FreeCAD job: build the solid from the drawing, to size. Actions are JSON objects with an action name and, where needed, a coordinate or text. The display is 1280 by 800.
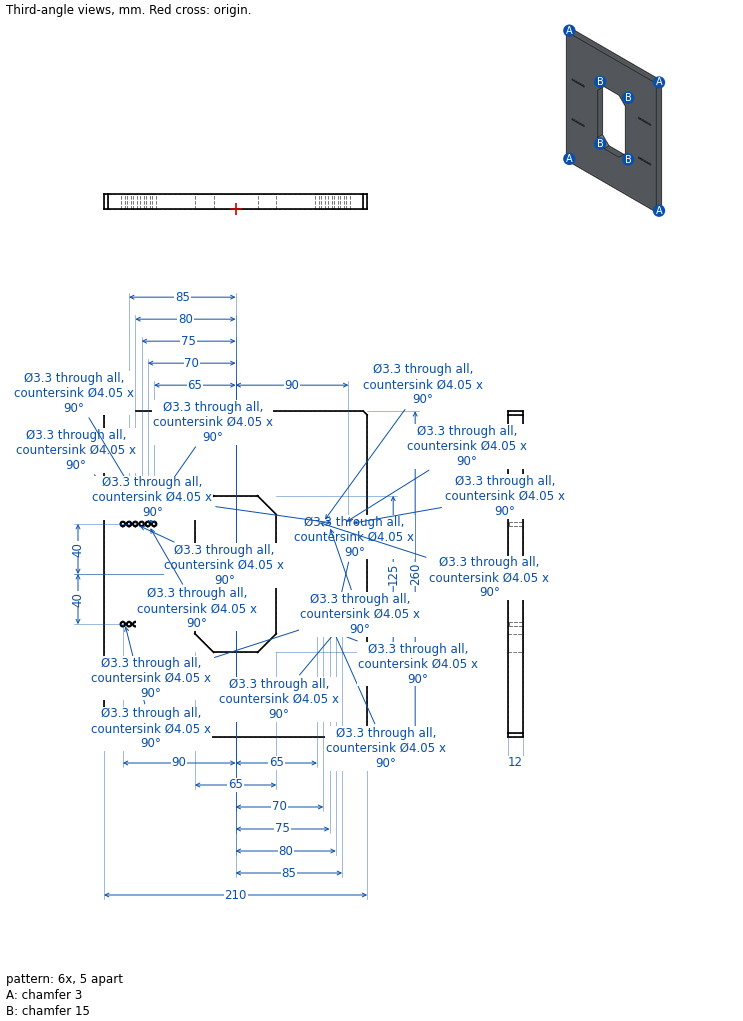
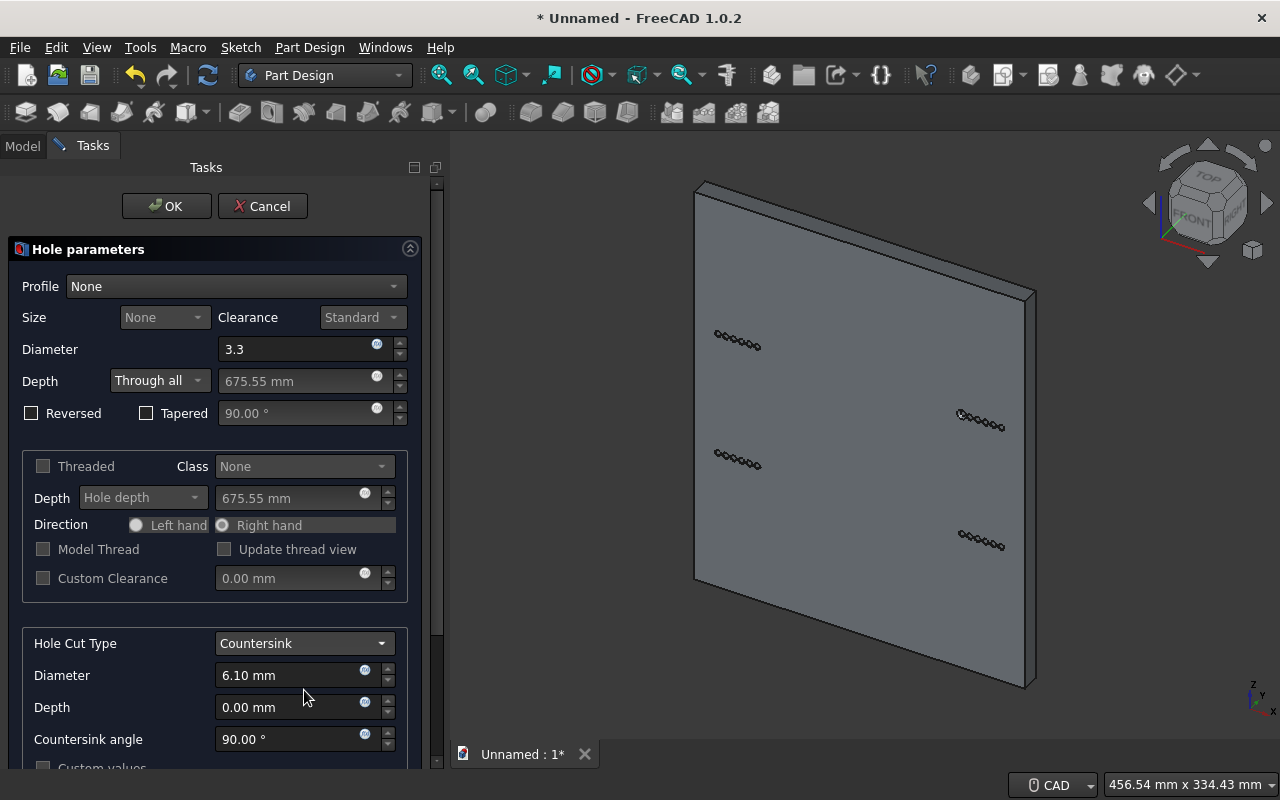
{"action": "triple_click", "coordinate": [298, 675]}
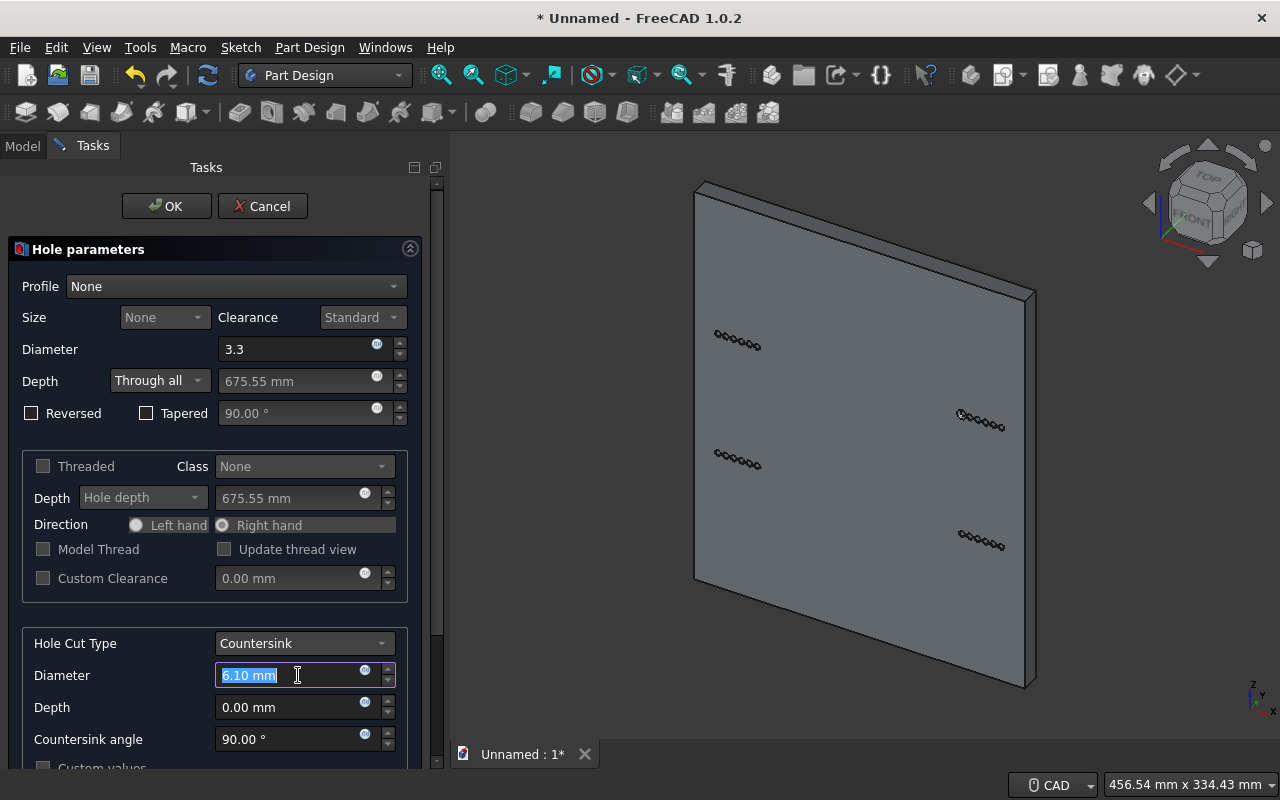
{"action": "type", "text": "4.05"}
{"action": "key", "text": "Tab"}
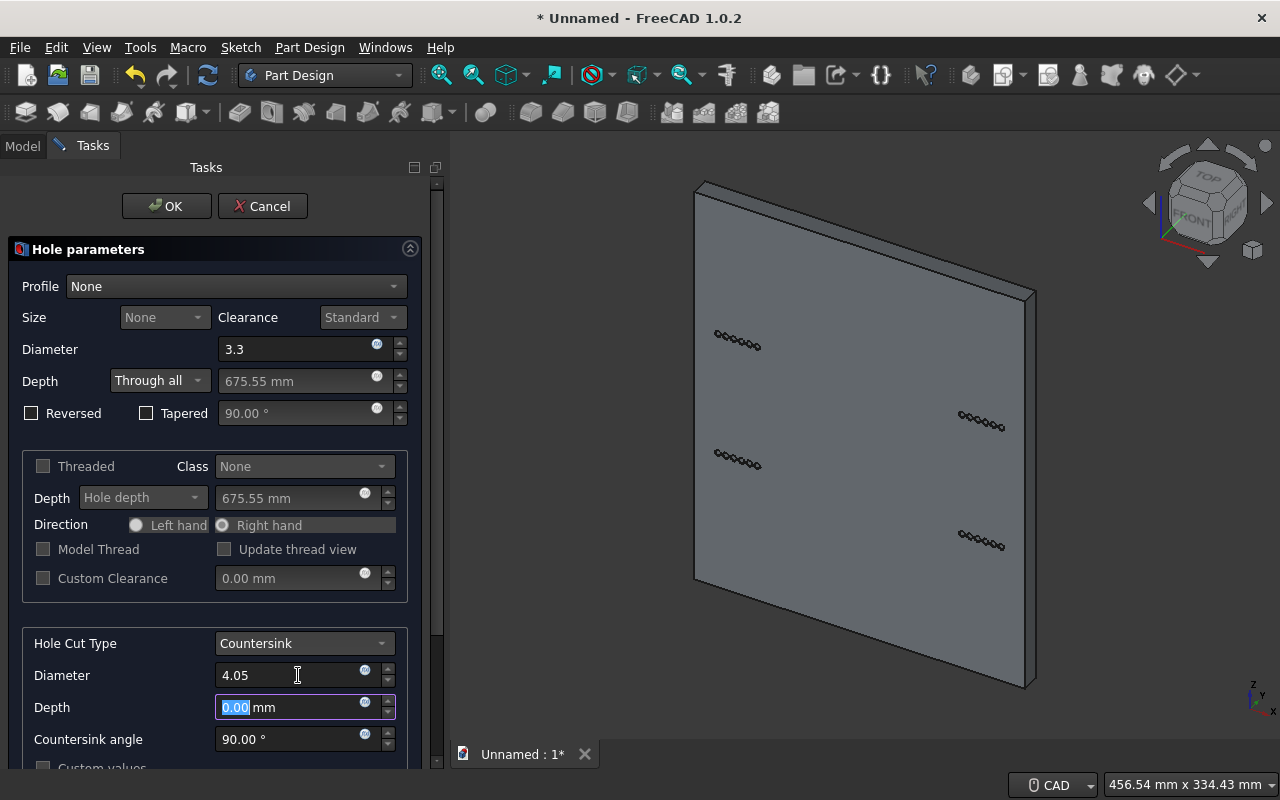
{"action": "left_click", "coordinate": [167, 206]}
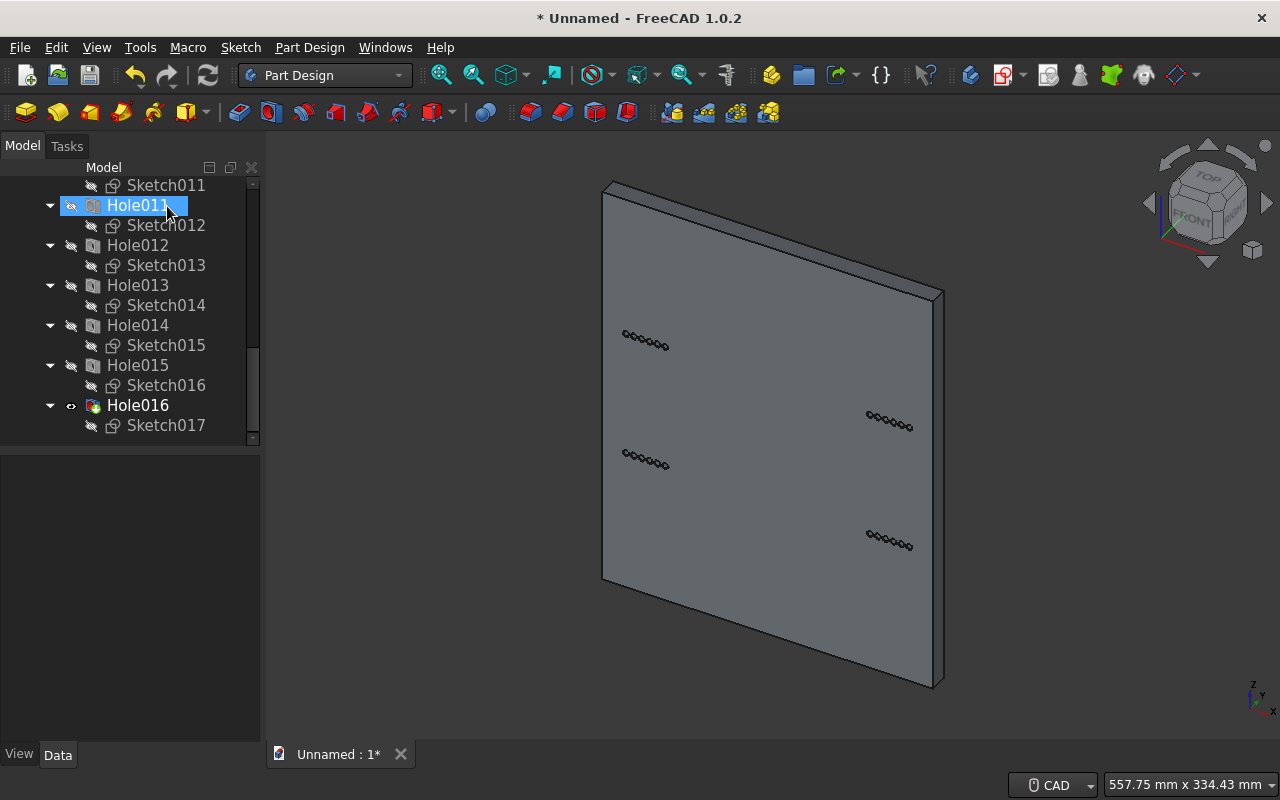
{"action": "left_click", "coordinate": [938, 295]}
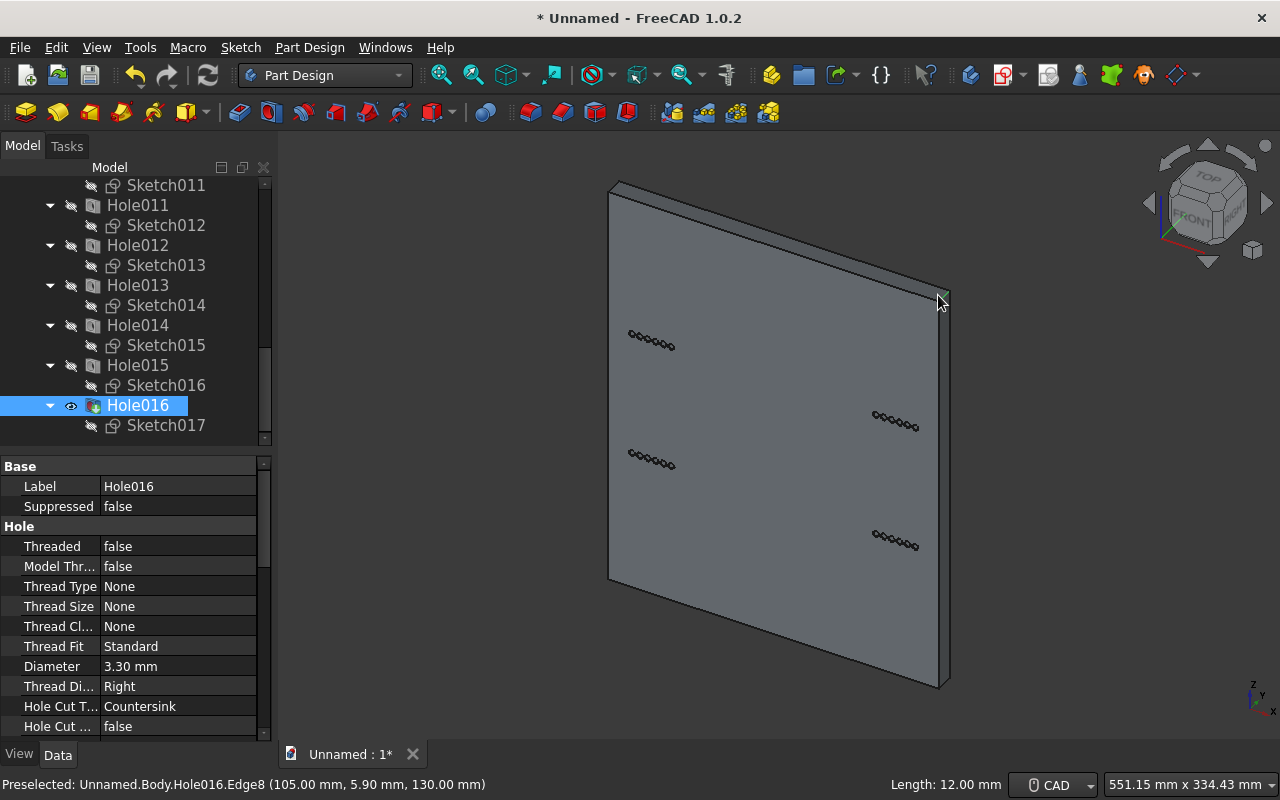
{"action": "scroll", "coordinate": [614, 186], "scroll_direction": "up", "scroll_amount": 4}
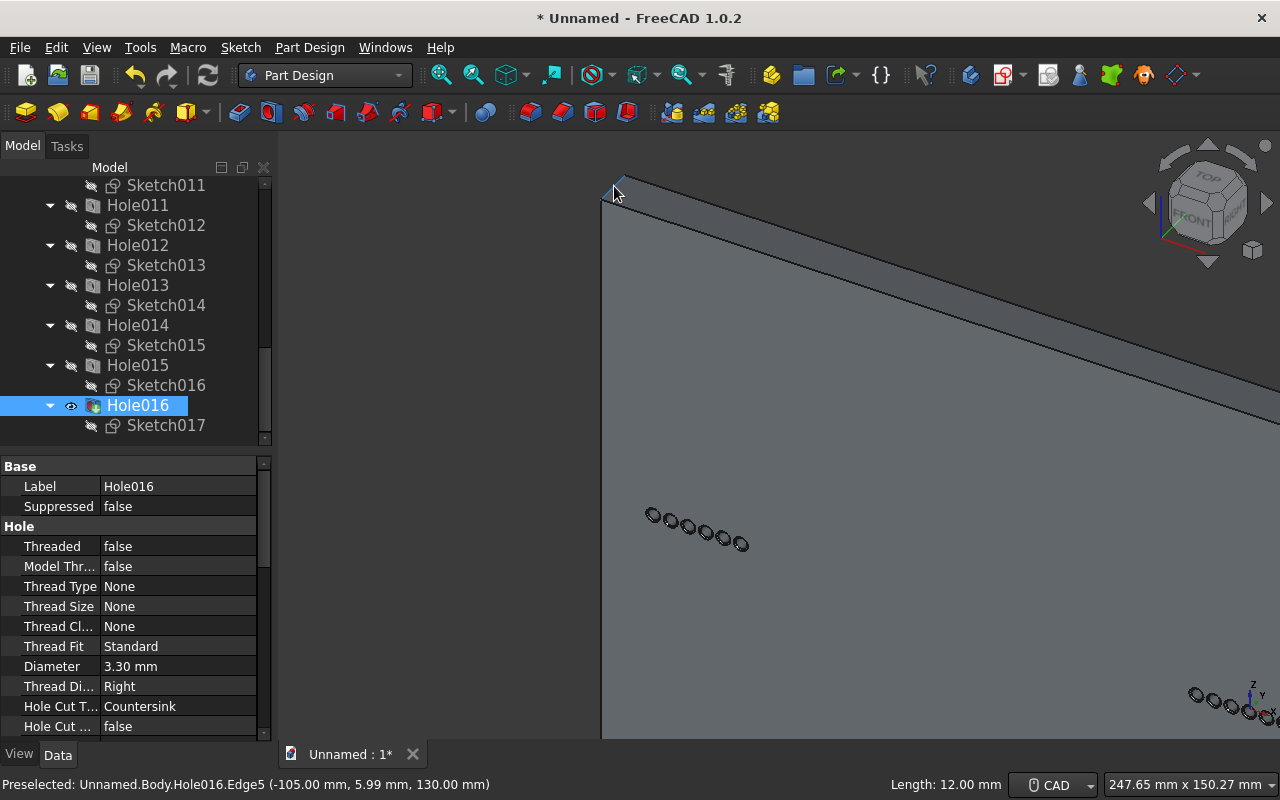
{"action": "left_click", "coordinate": [442, 76]}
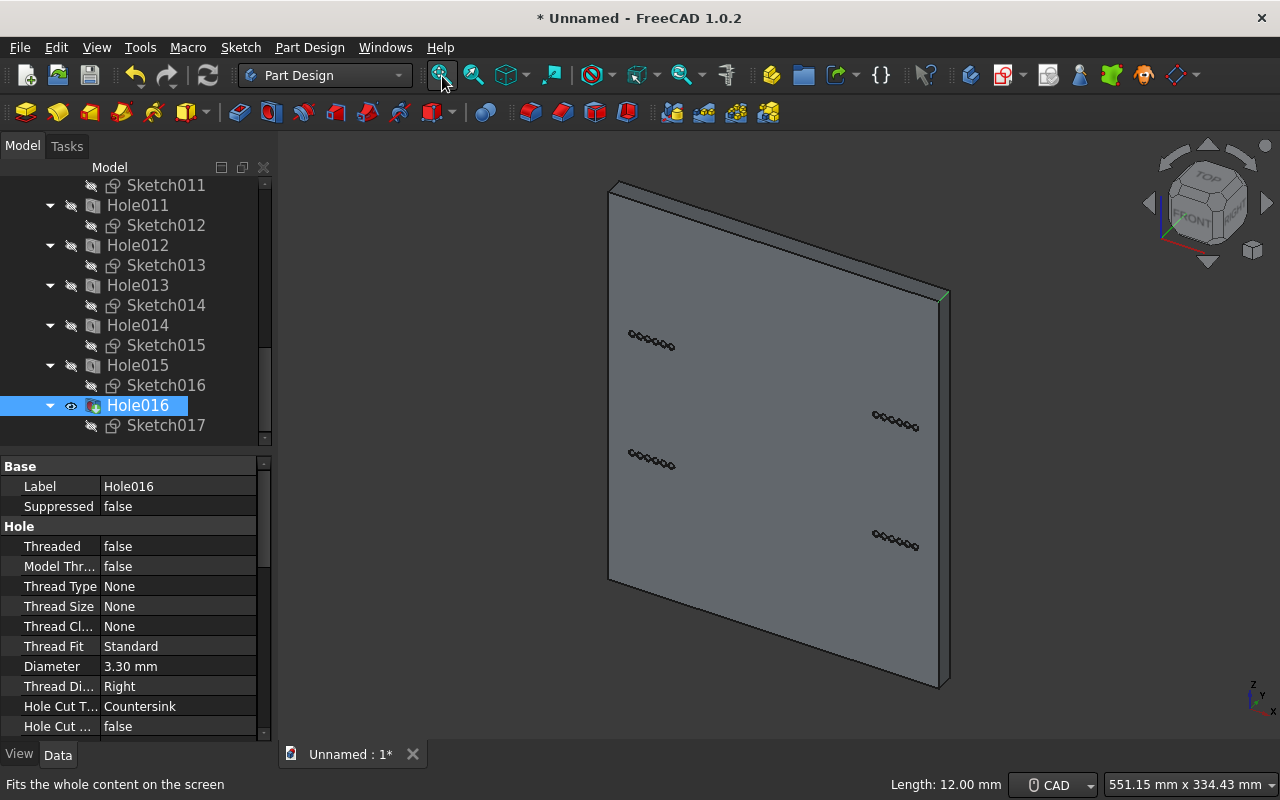
{"action": "key", "text": "0"}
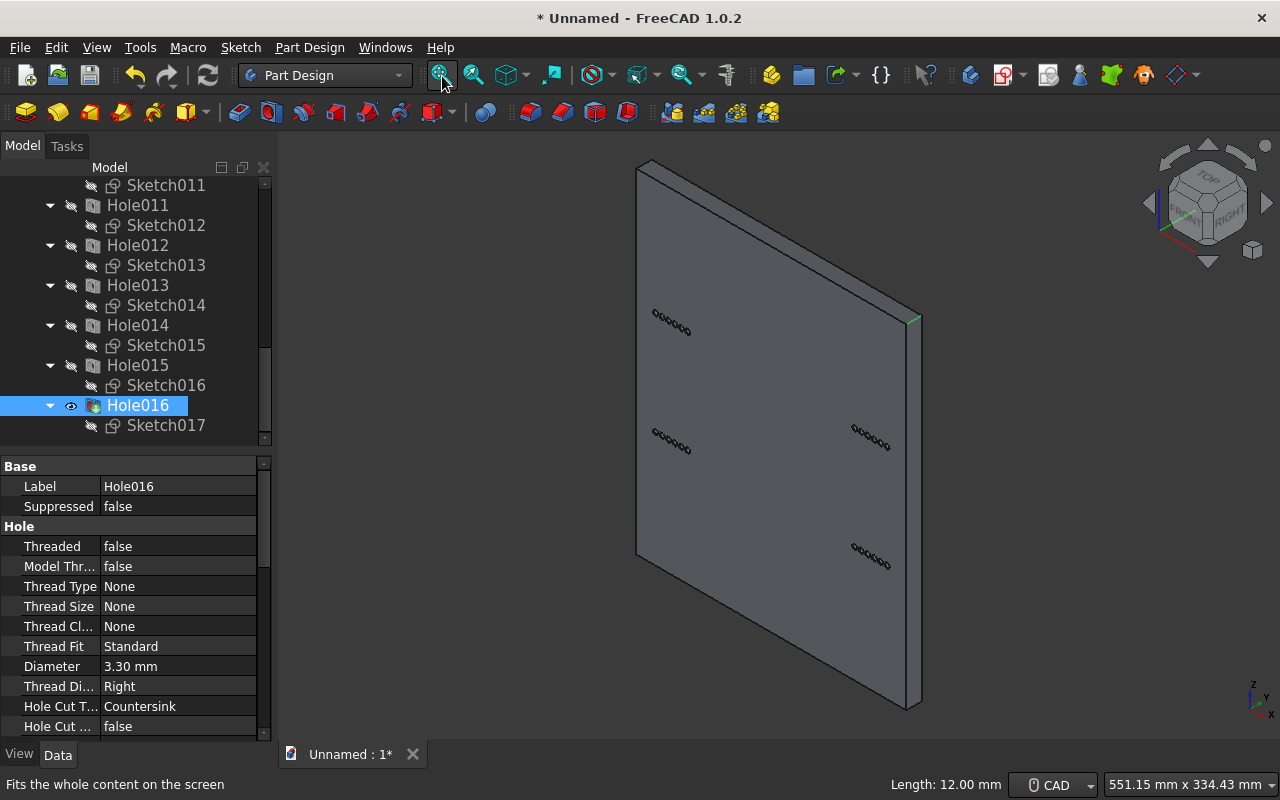
{"action": "scroll", "coordinate": [644, 163], "scroll_direction": "up", "scroll_amount": 4}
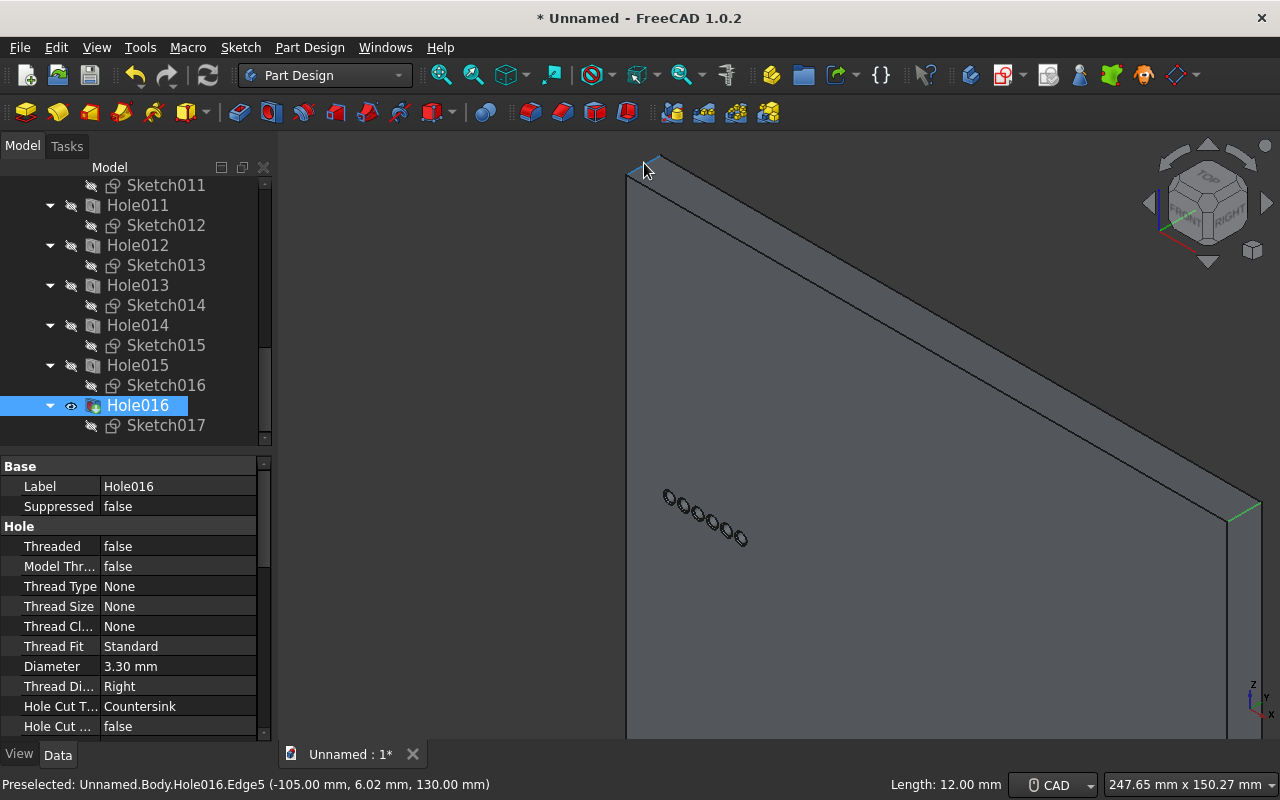
{"action": "left_click", "coordinate": [442, 76]}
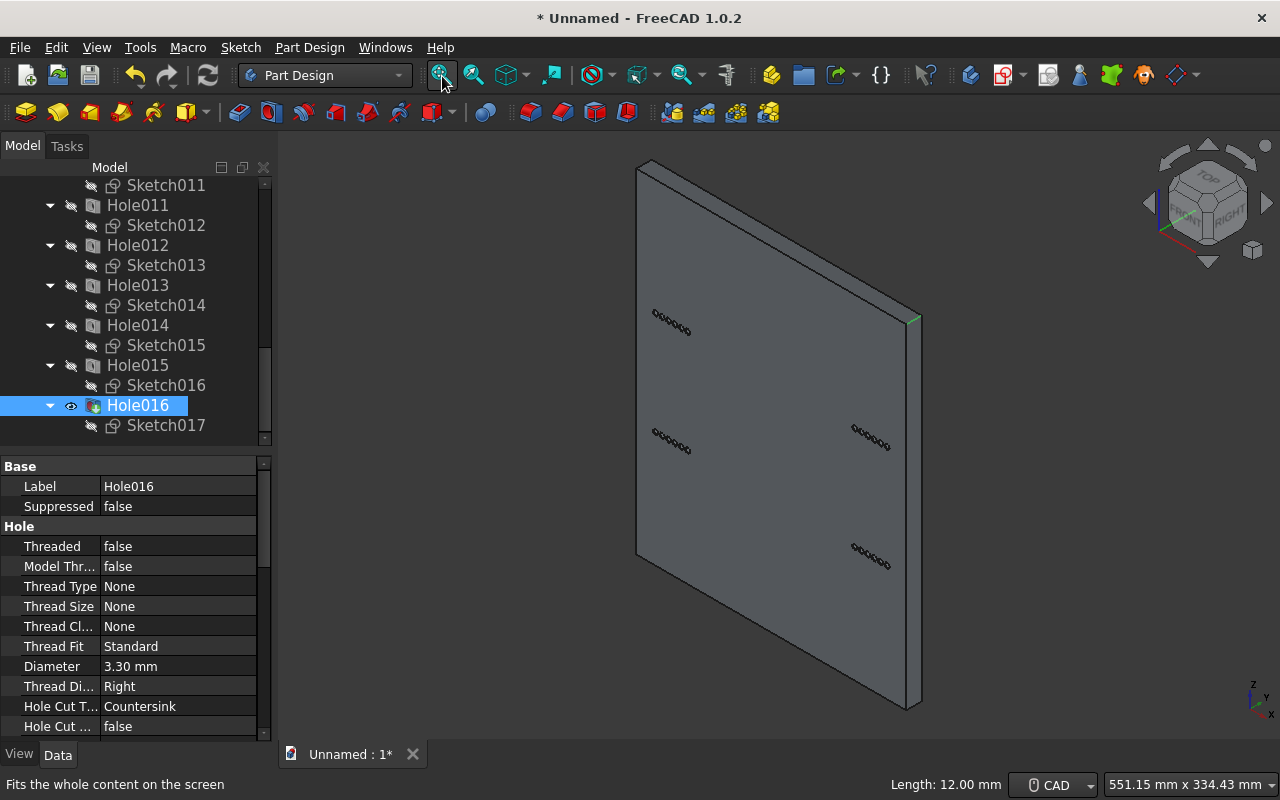
{"action": "key", "text": "2"}